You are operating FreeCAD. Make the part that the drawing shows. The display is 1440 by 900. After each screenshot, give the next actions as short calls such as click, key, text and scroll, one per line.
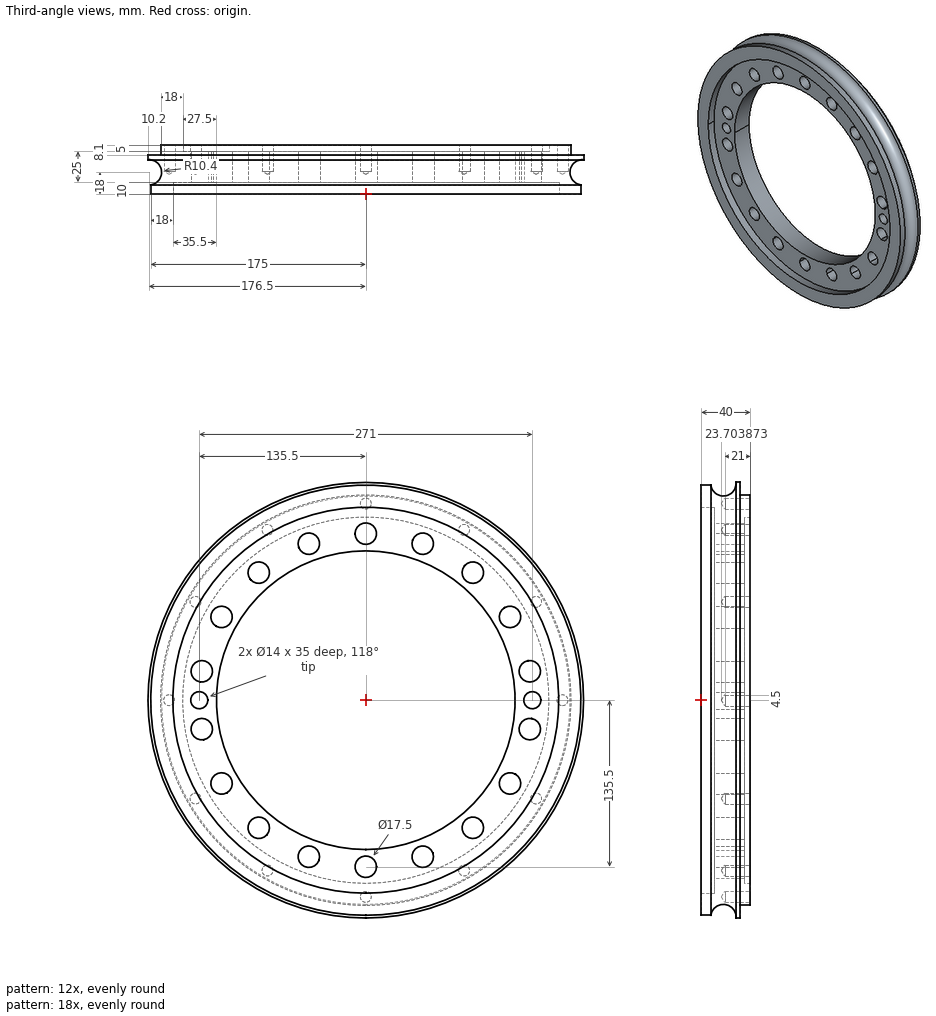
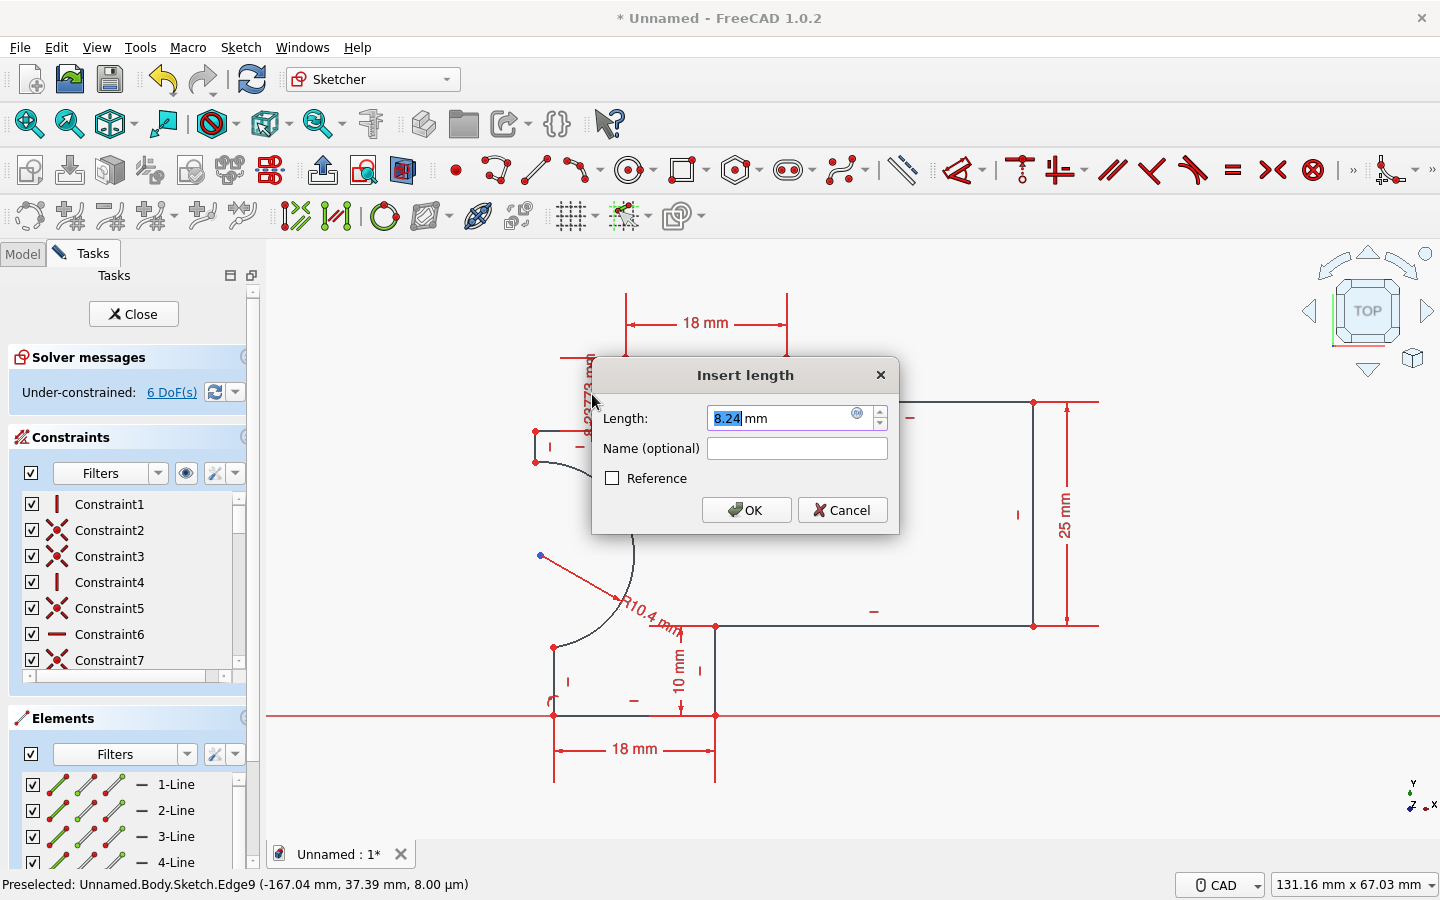
text(8.1)
key(Return)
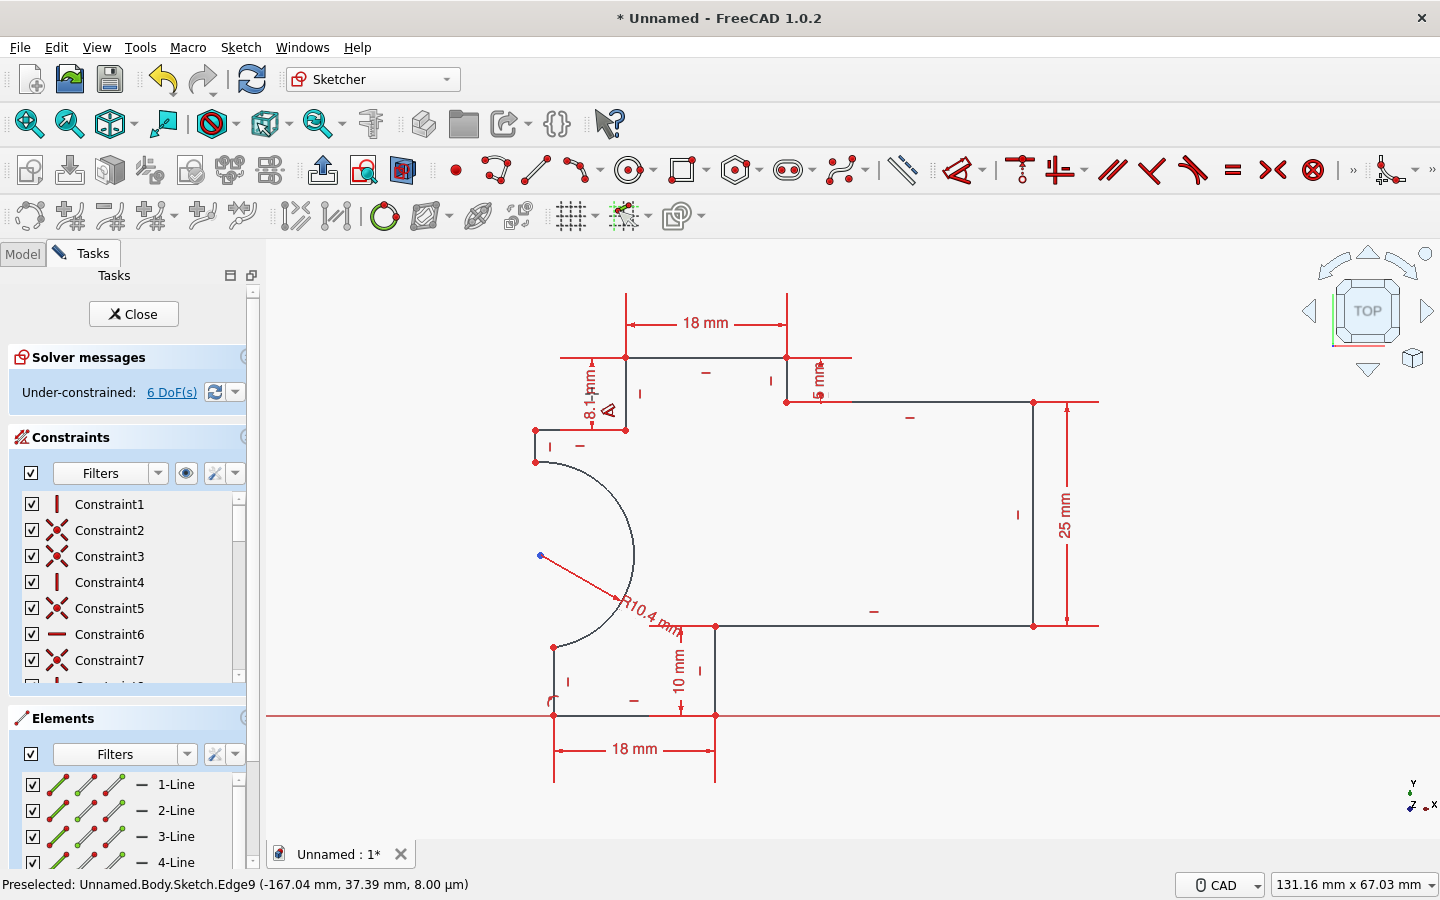
click(541, 555)
click(507, 635)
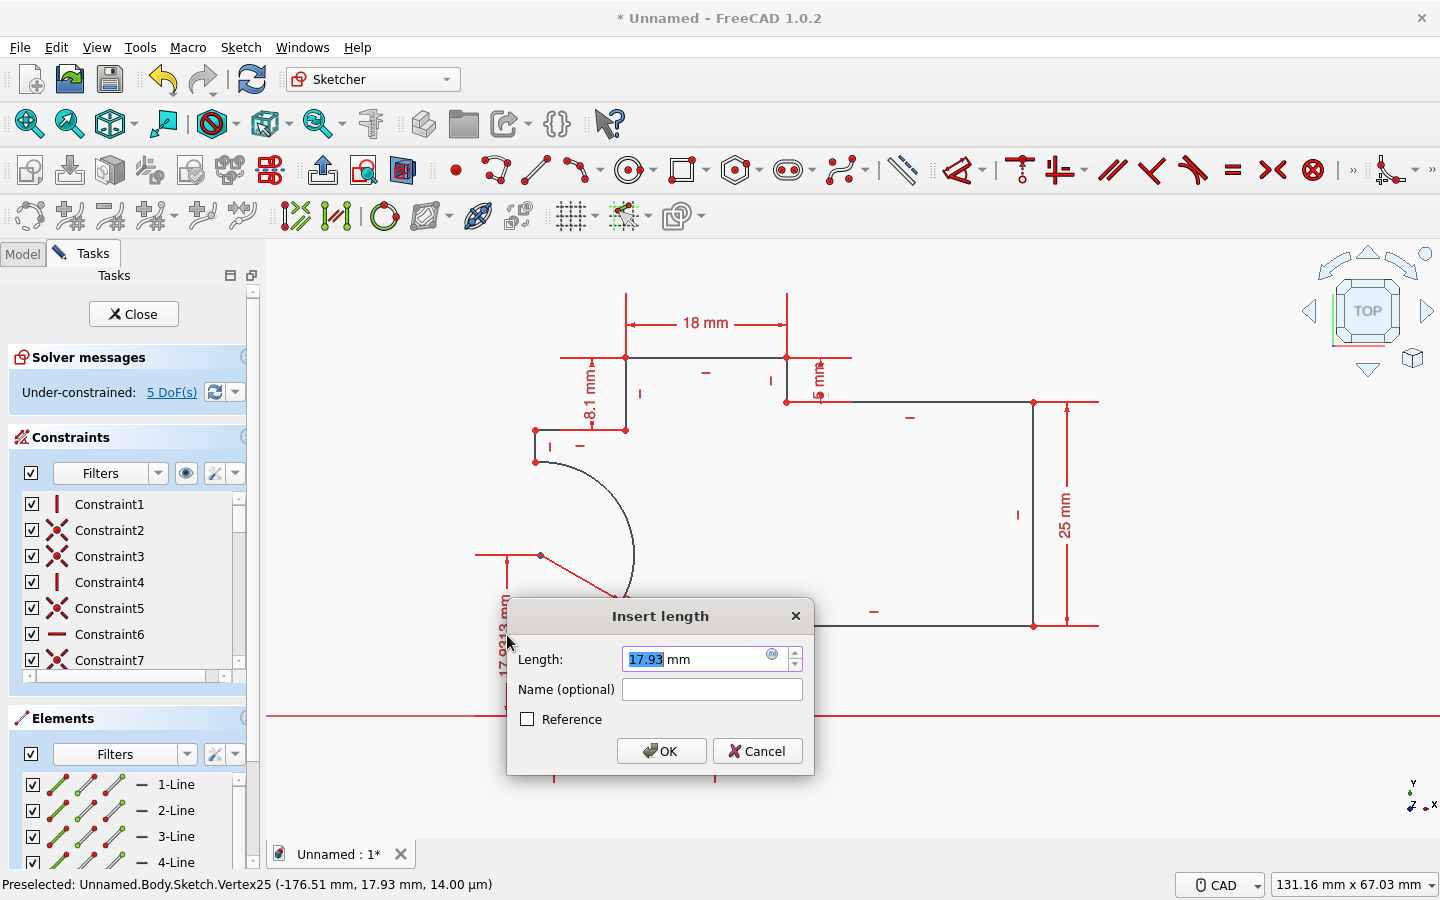
text(18)
key(Return)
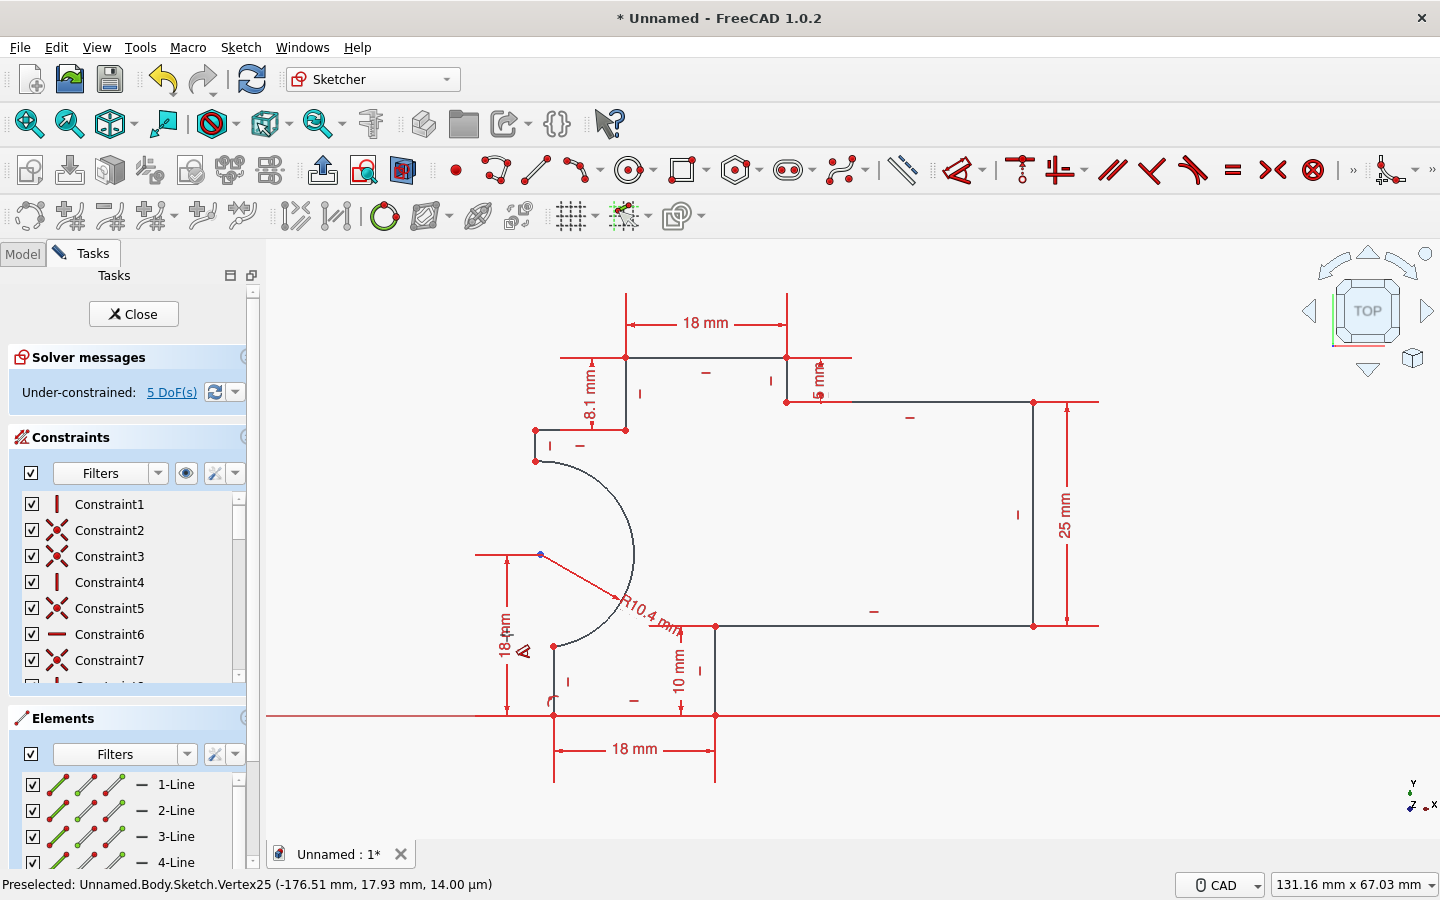
click(811, 626)
click(874, 660)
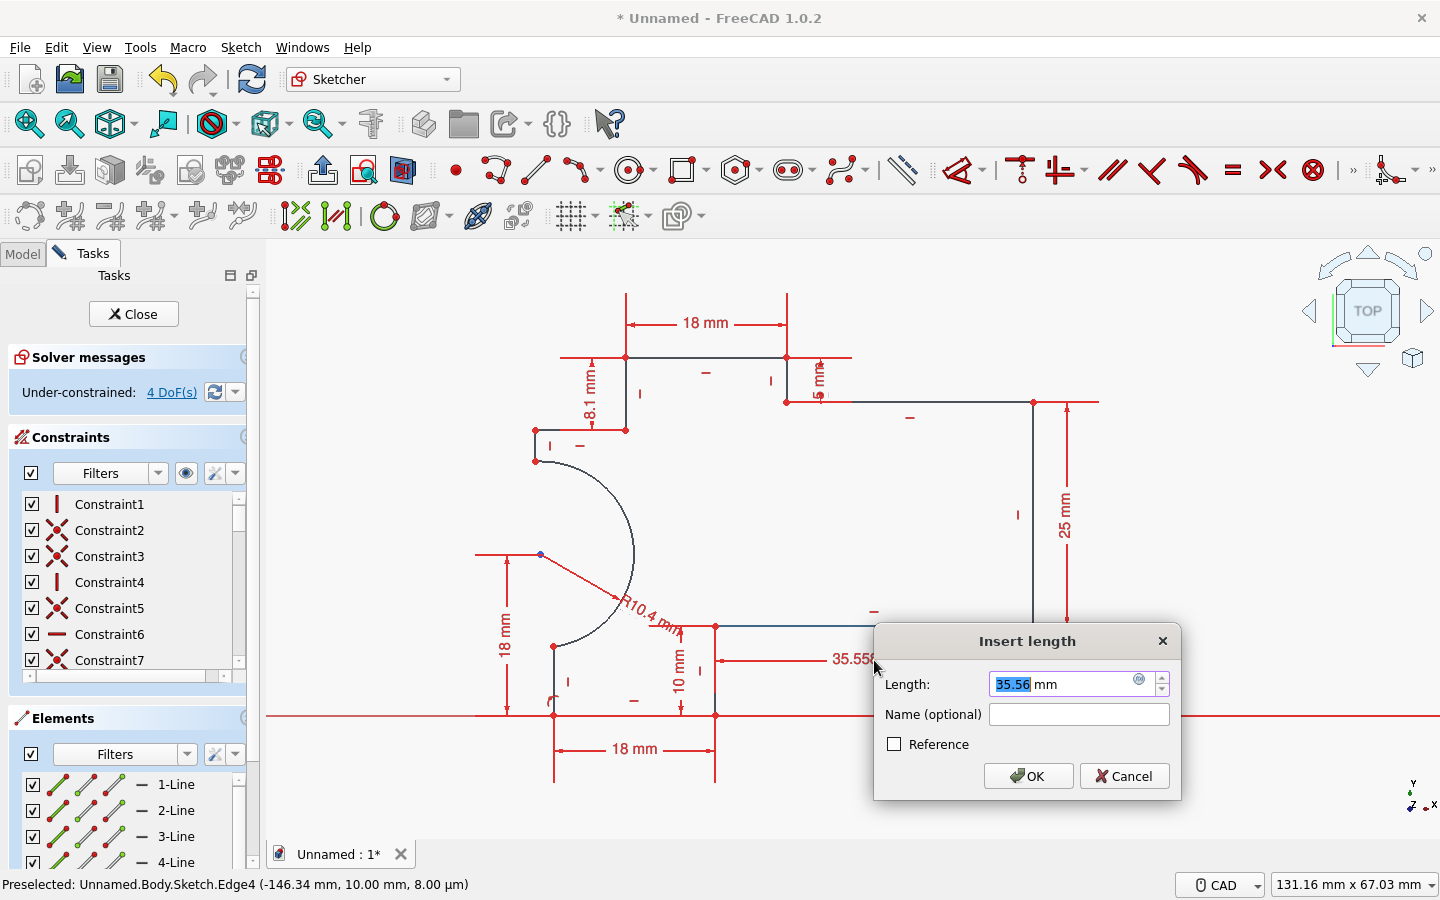
text(35.5)
key(Return)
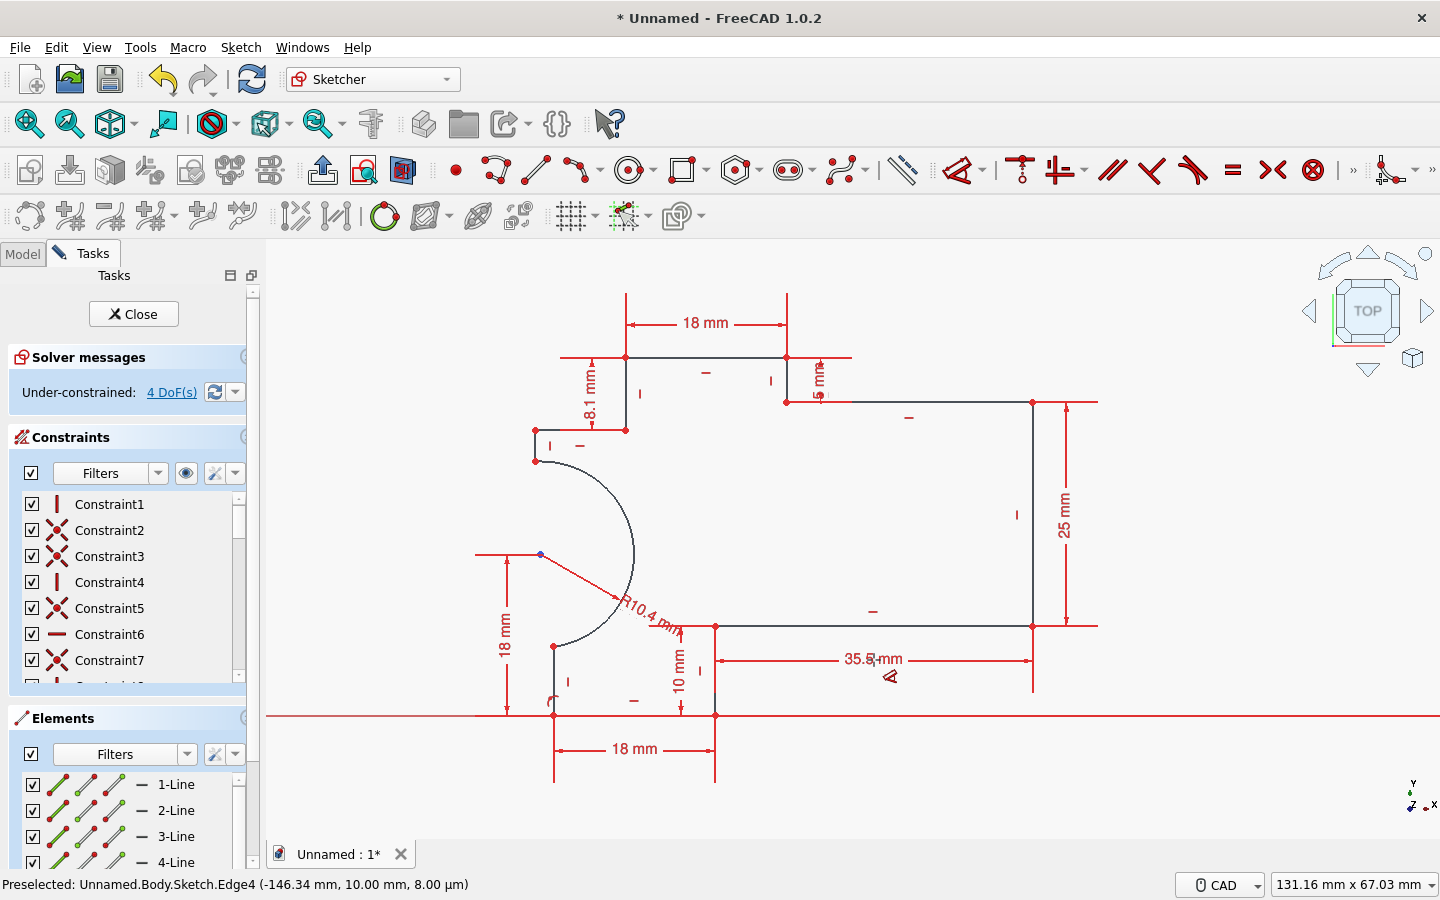
click(959, 402)
click(910, 368)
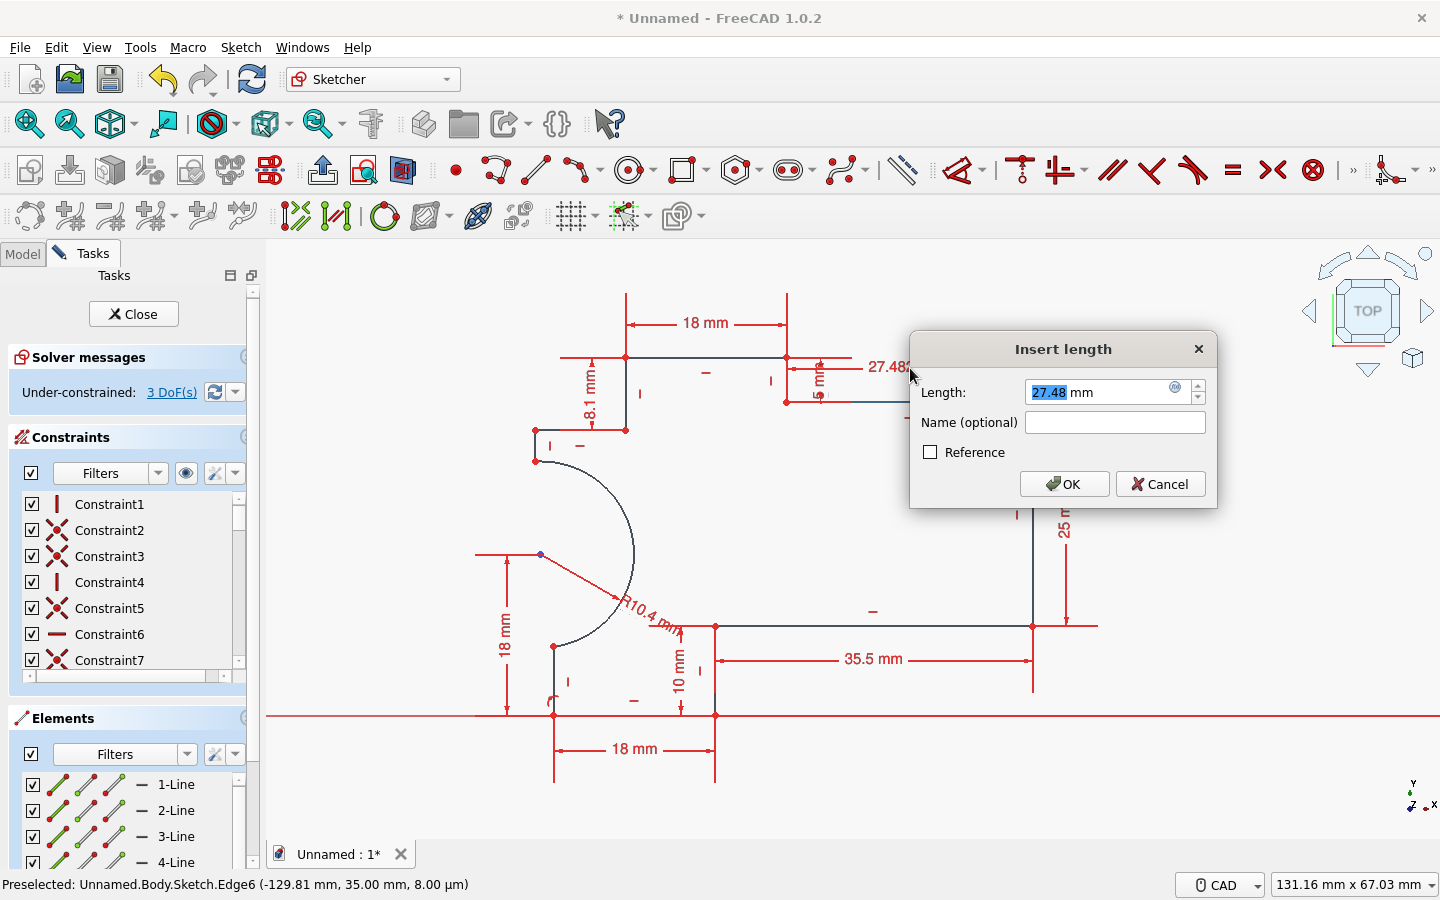
text(27.5)
key(Return)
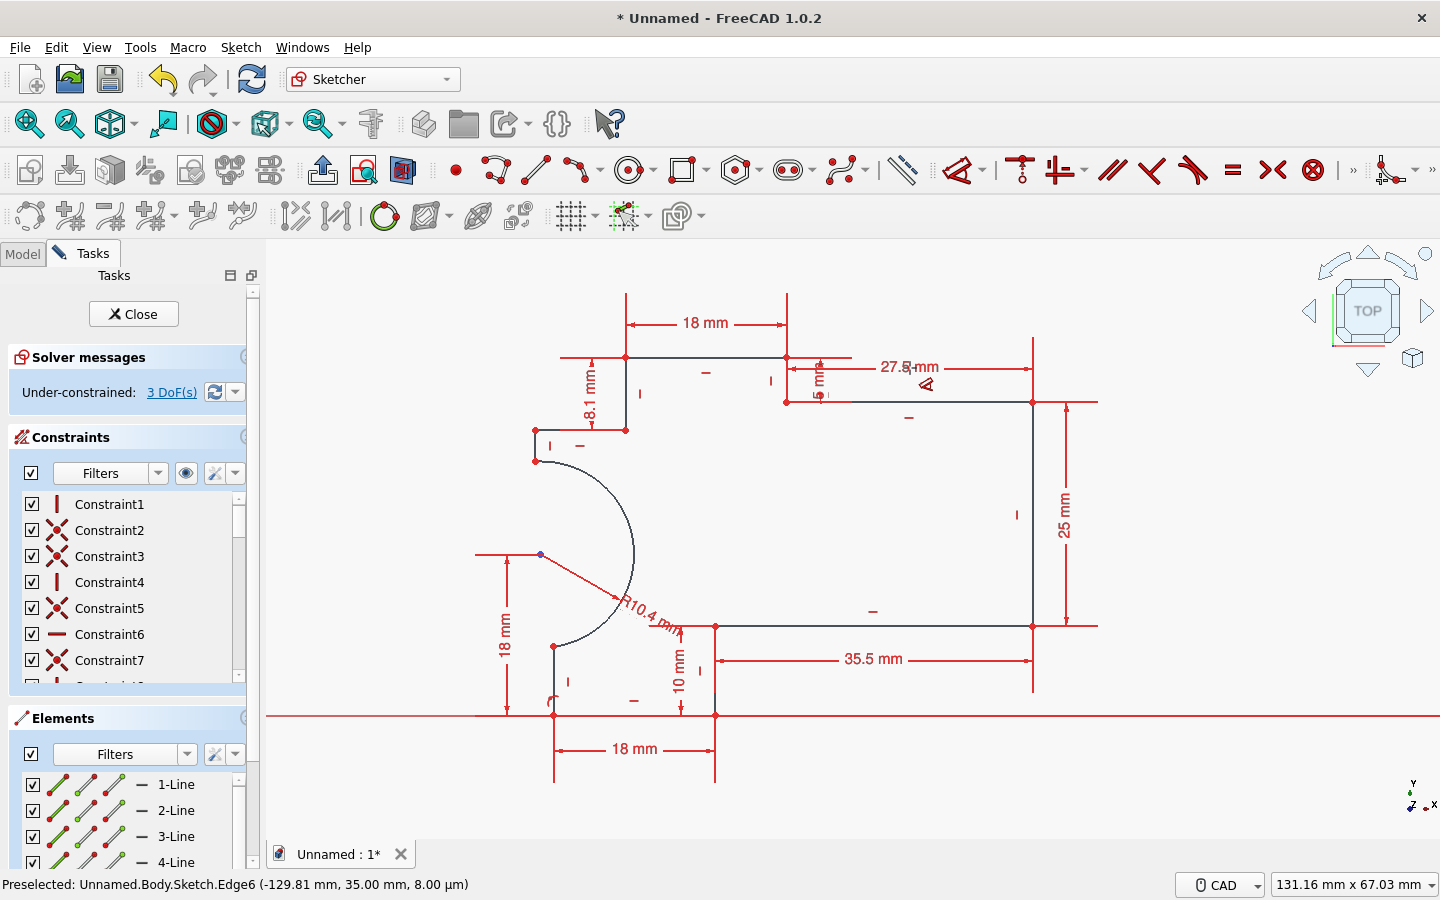
click(598, 430)
click(601, 464)